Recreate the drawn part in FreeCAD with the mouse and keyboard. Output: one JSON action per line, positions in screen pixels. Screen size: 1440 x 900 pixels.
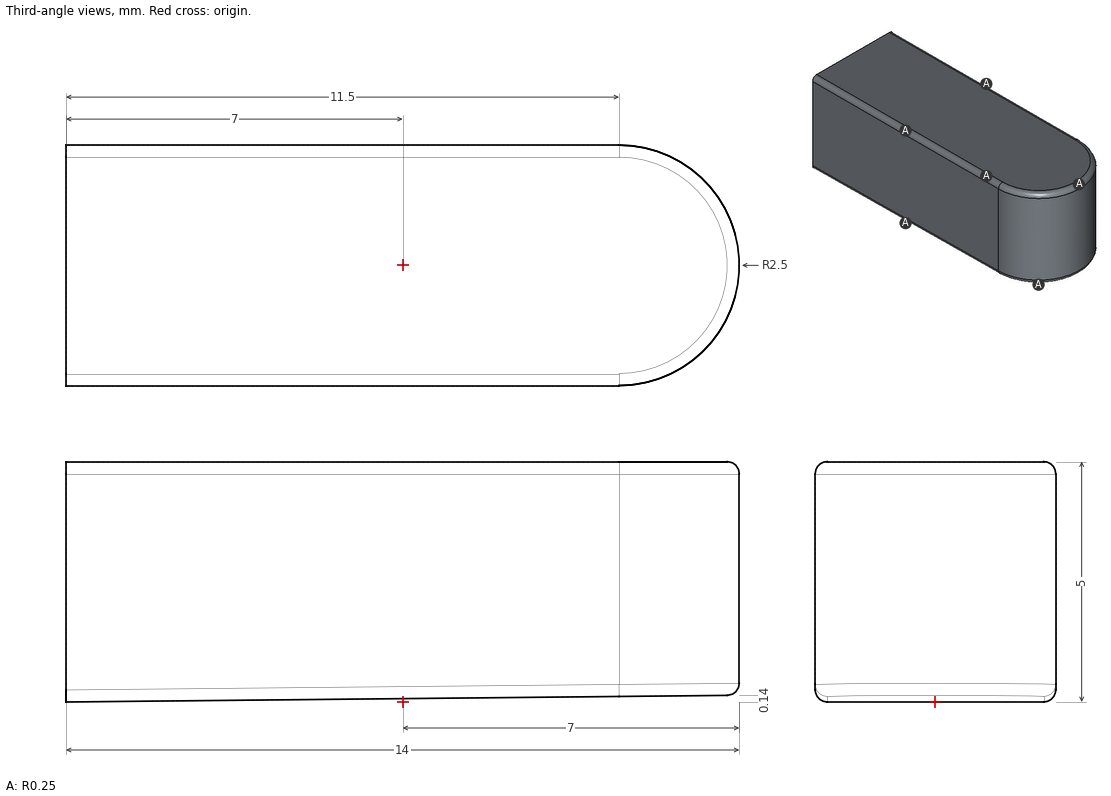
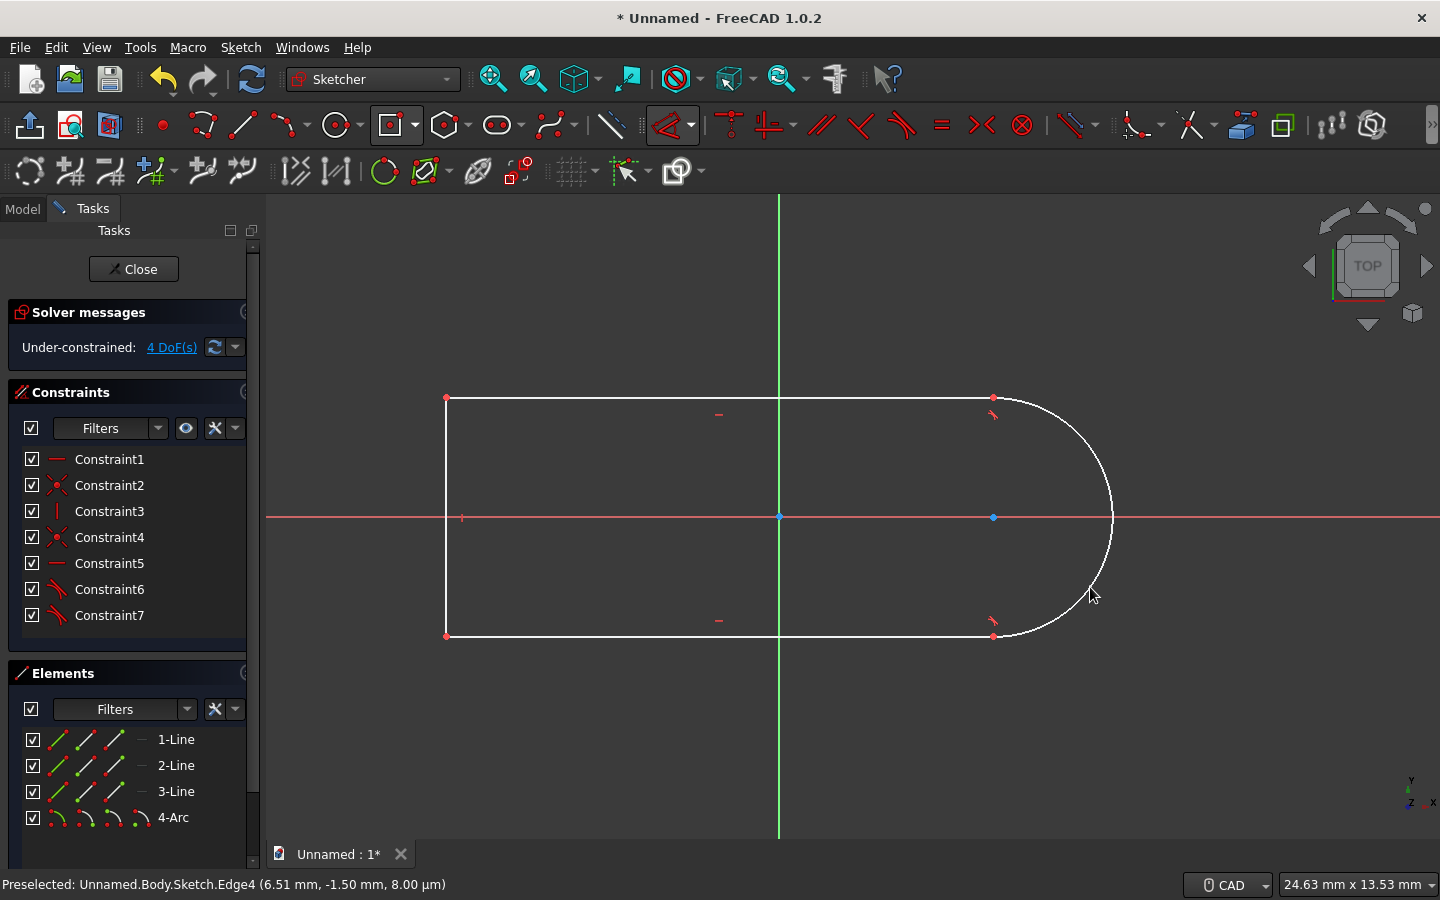
{"action": "left_click", "coordinate": [993, 517]}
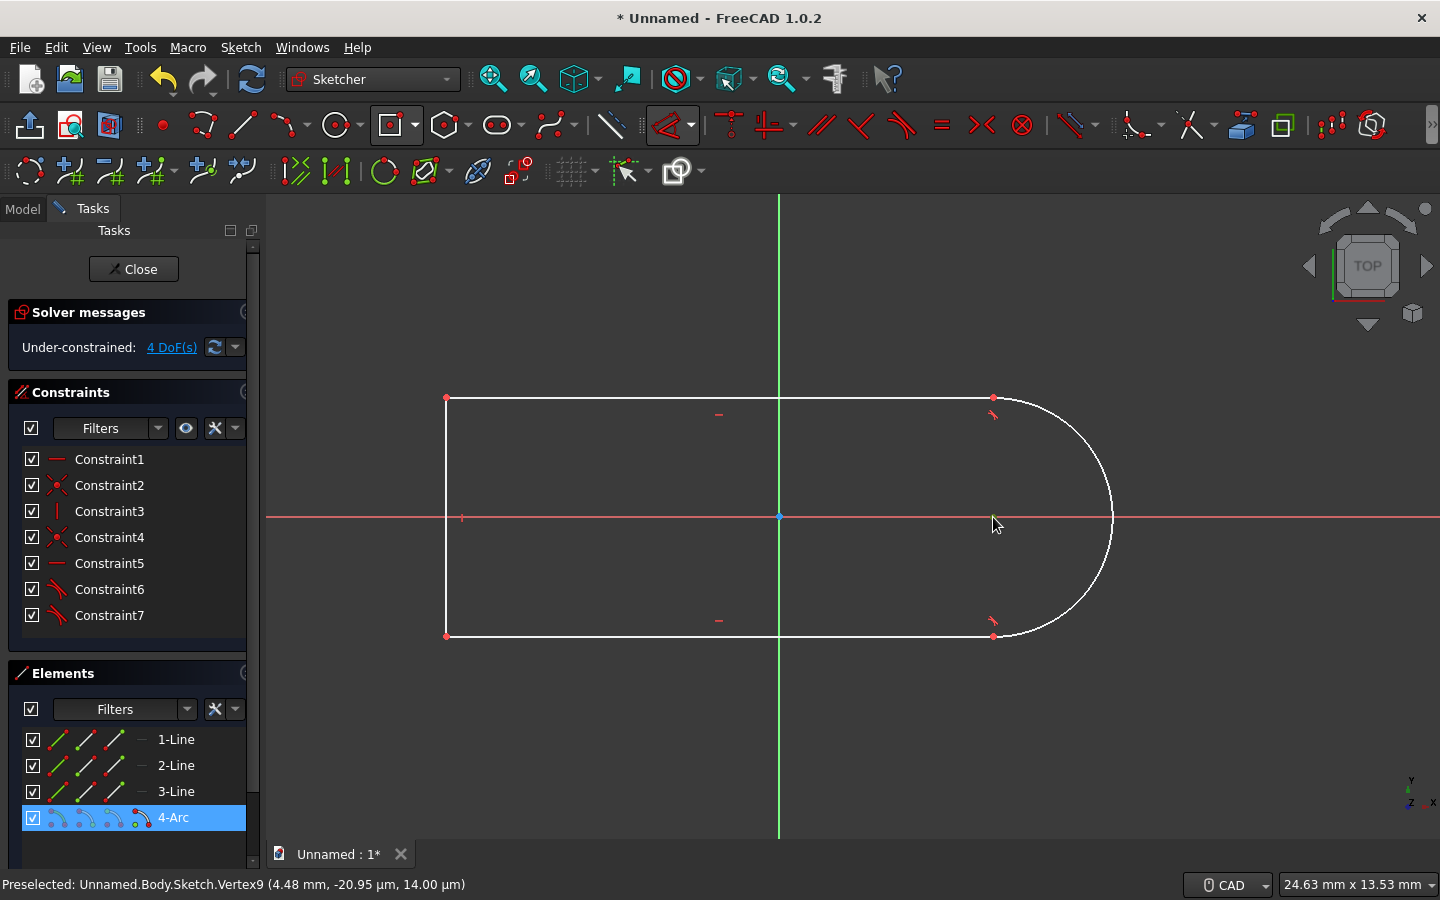
{"action": "left_click", "coordinate": [364, 516]}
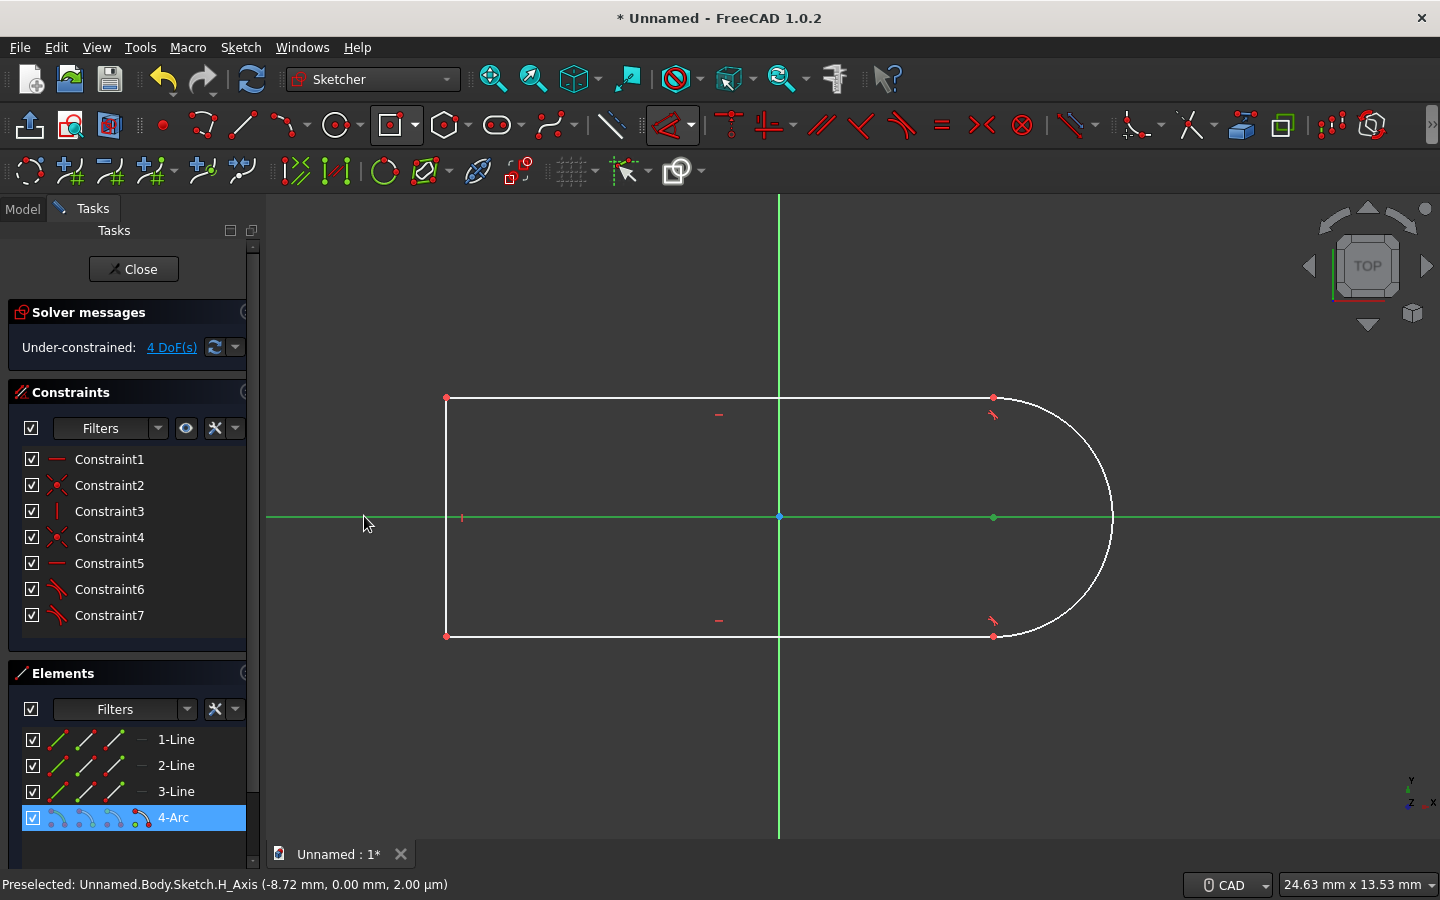
{"action": "left_click", "coordinate": [730, 126]}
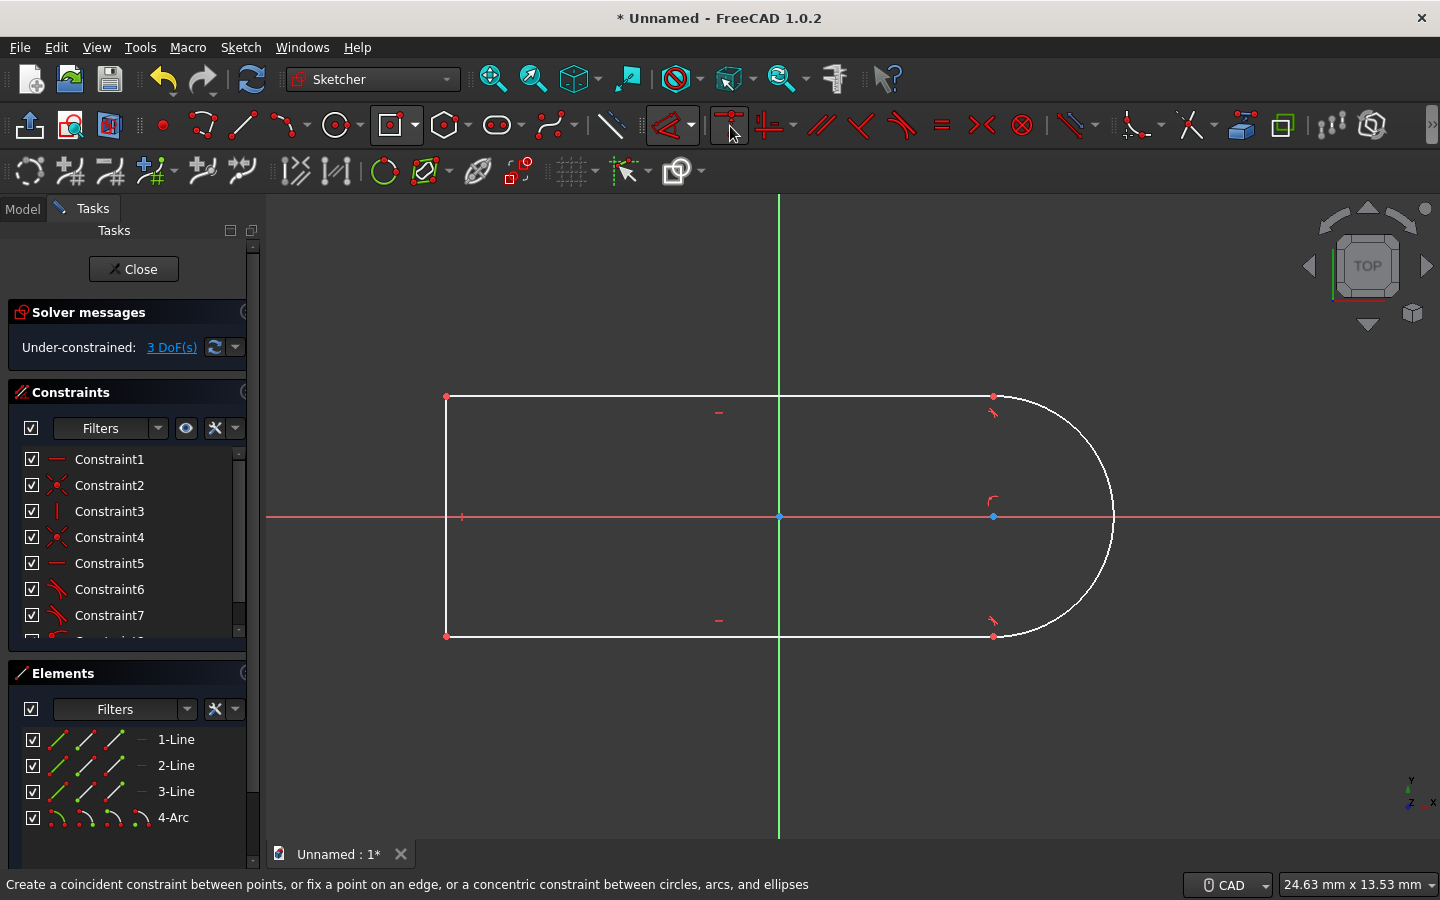
{"action": "key", "text": "d"}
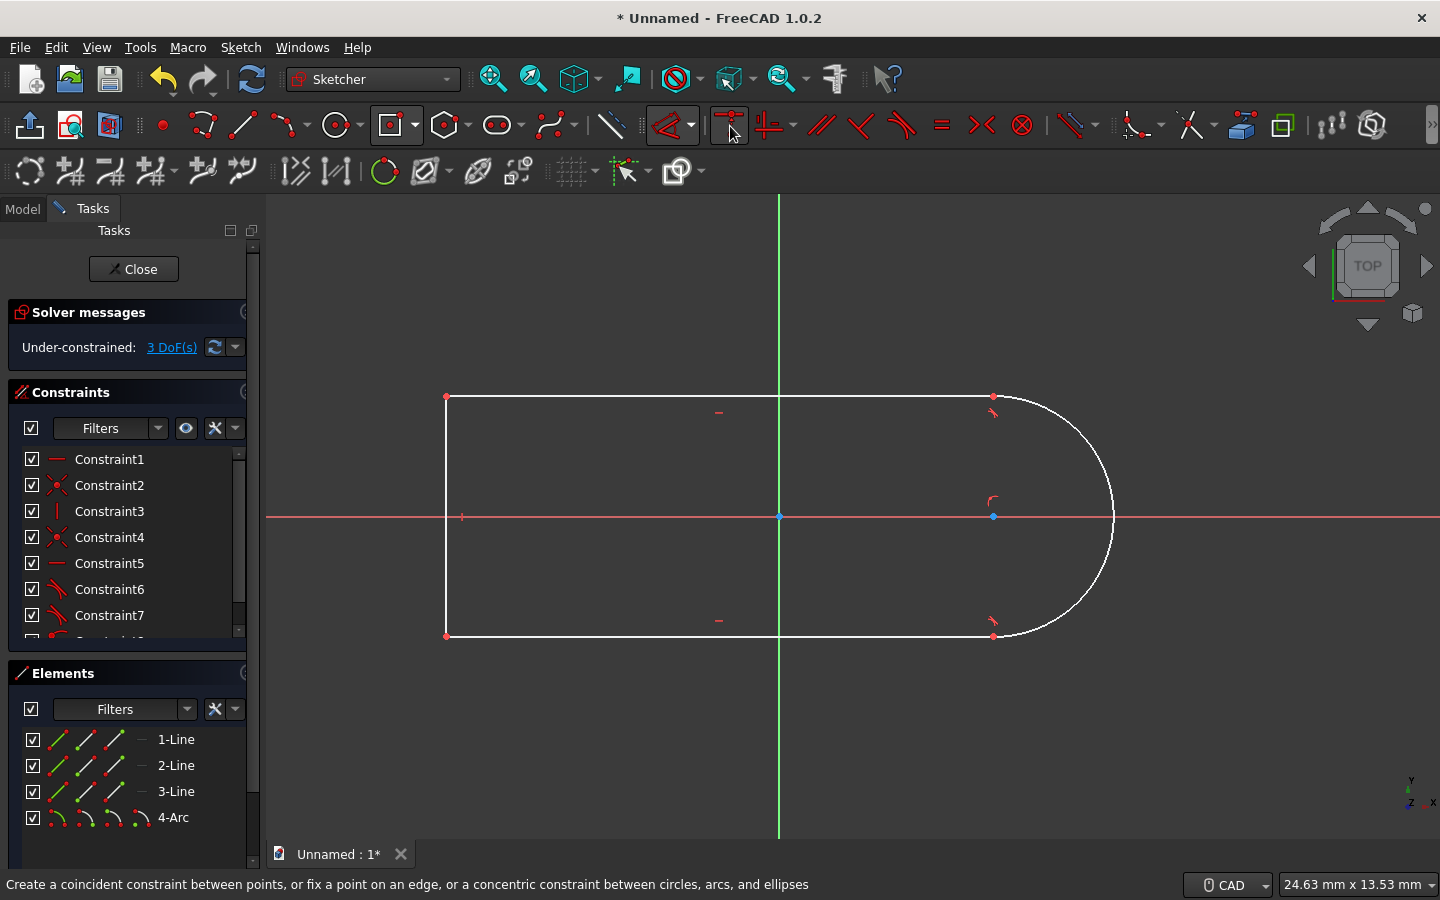
{"action": "left_click", "coordinate": [1091, 587]}
{"action": "left_click", "coordinate": [1117, 606]}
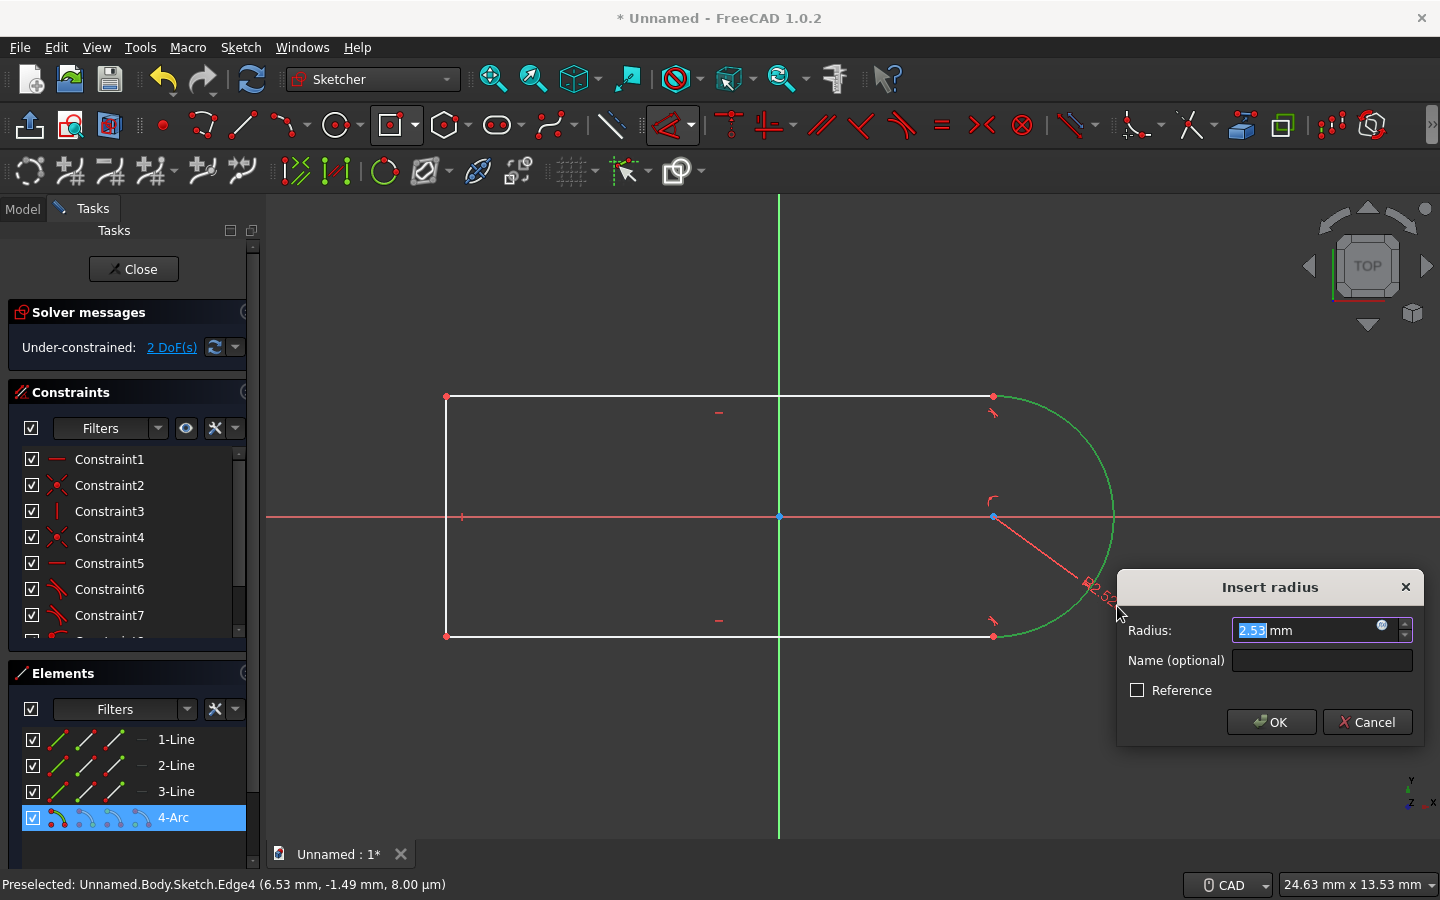
{"action": "type", "text": "2.5"}
{"action": "key", "text": "Return"}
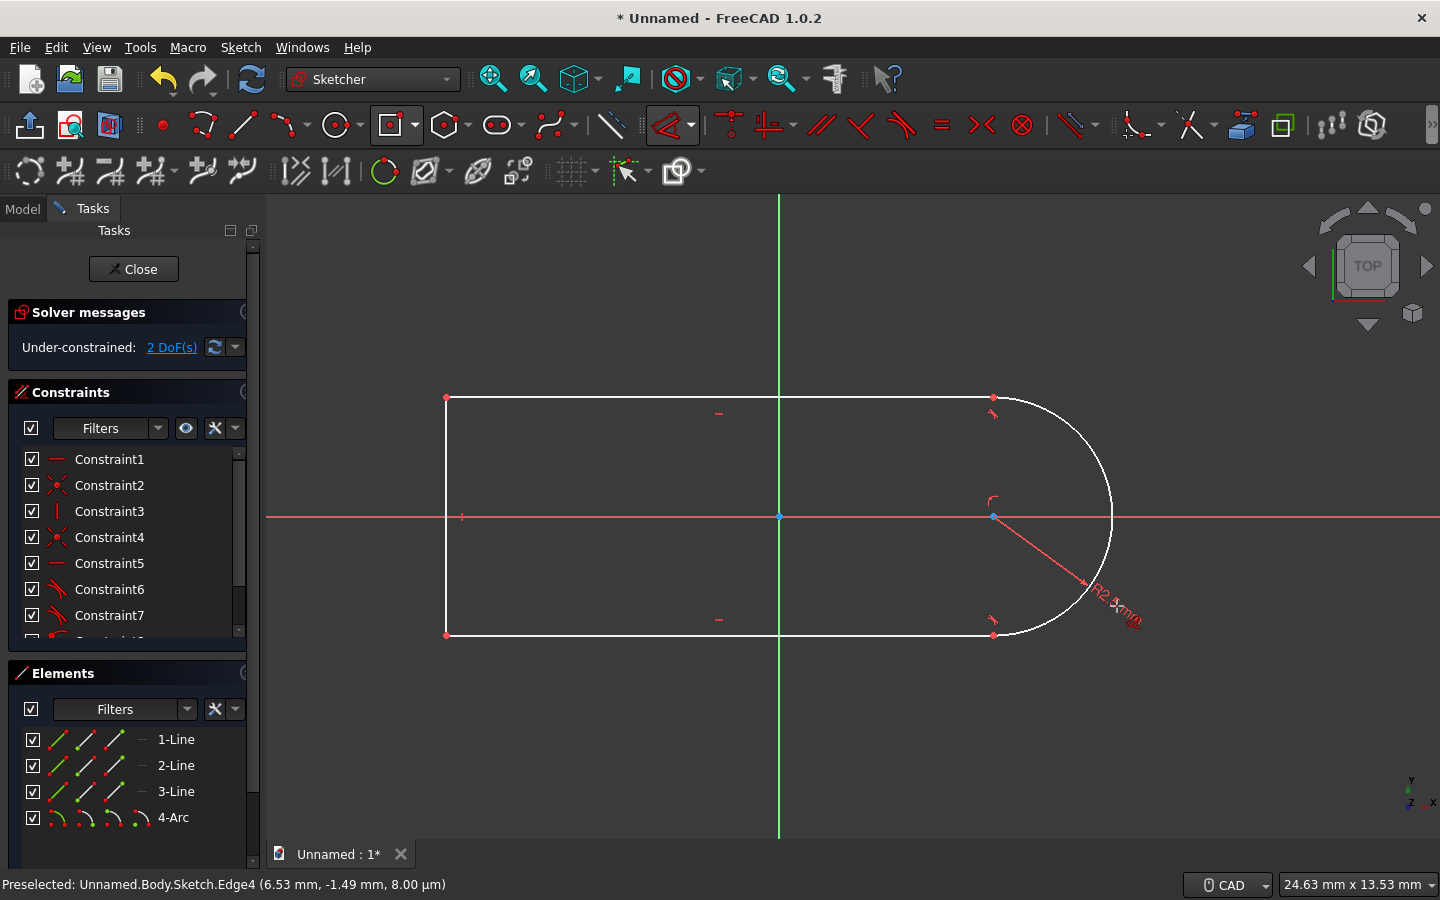
{"action": "left_click", "coordinate": [446, 397]}
{"action": "left_click", "coordinate": [613, 363]}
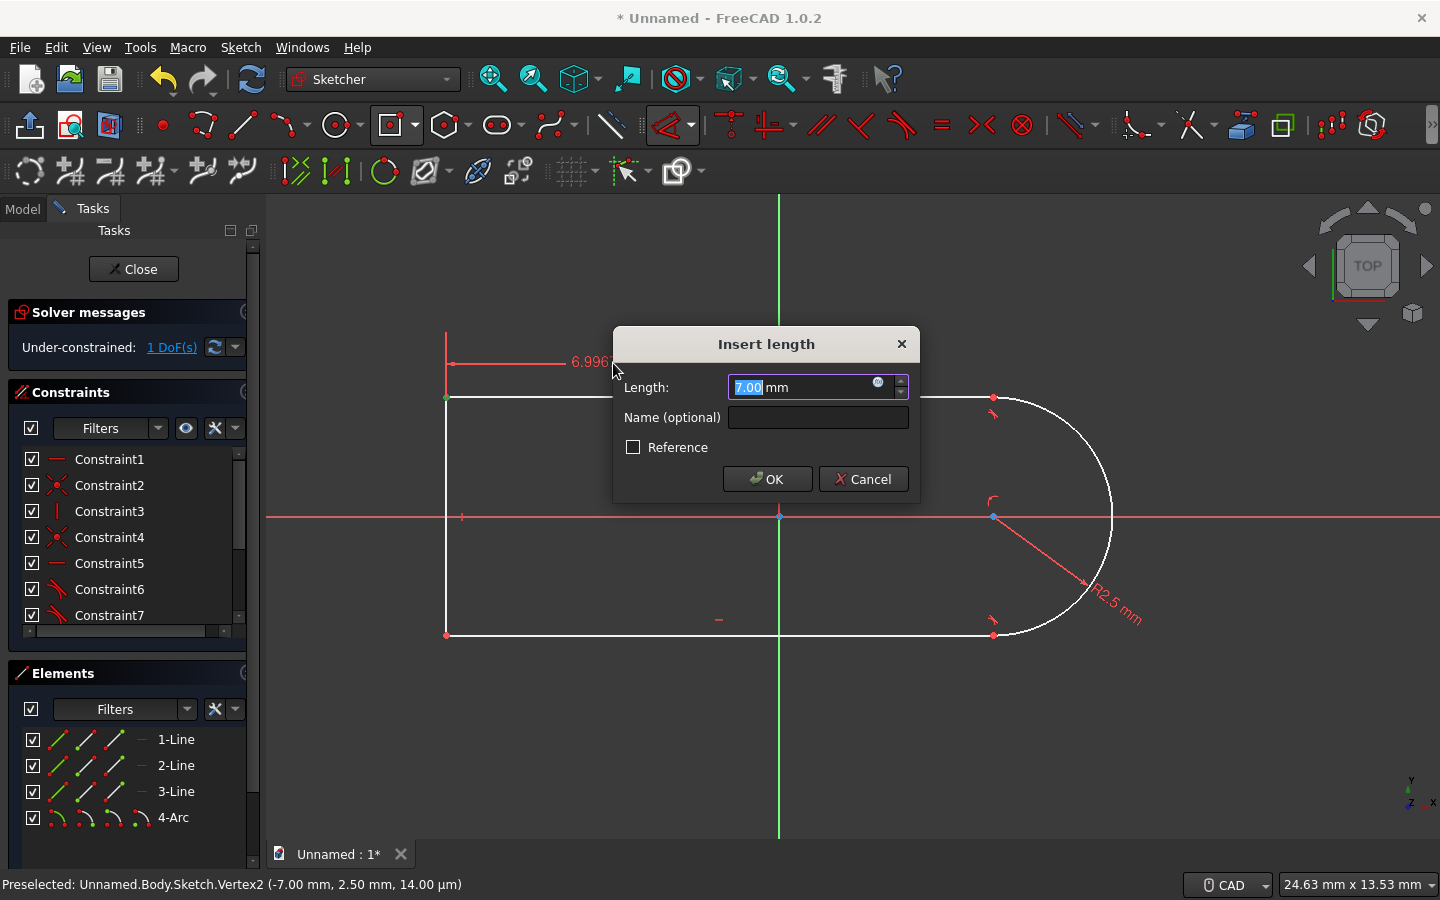
{"action": "type", "text": "7"}
{"action": "key", "text": "Return"}